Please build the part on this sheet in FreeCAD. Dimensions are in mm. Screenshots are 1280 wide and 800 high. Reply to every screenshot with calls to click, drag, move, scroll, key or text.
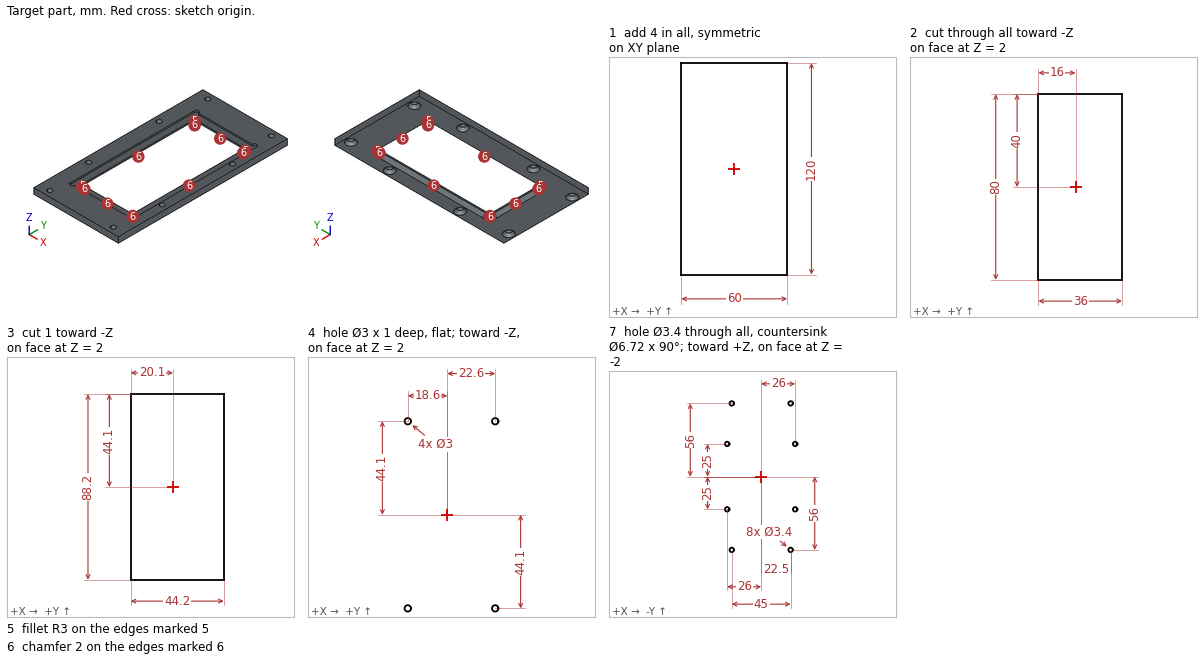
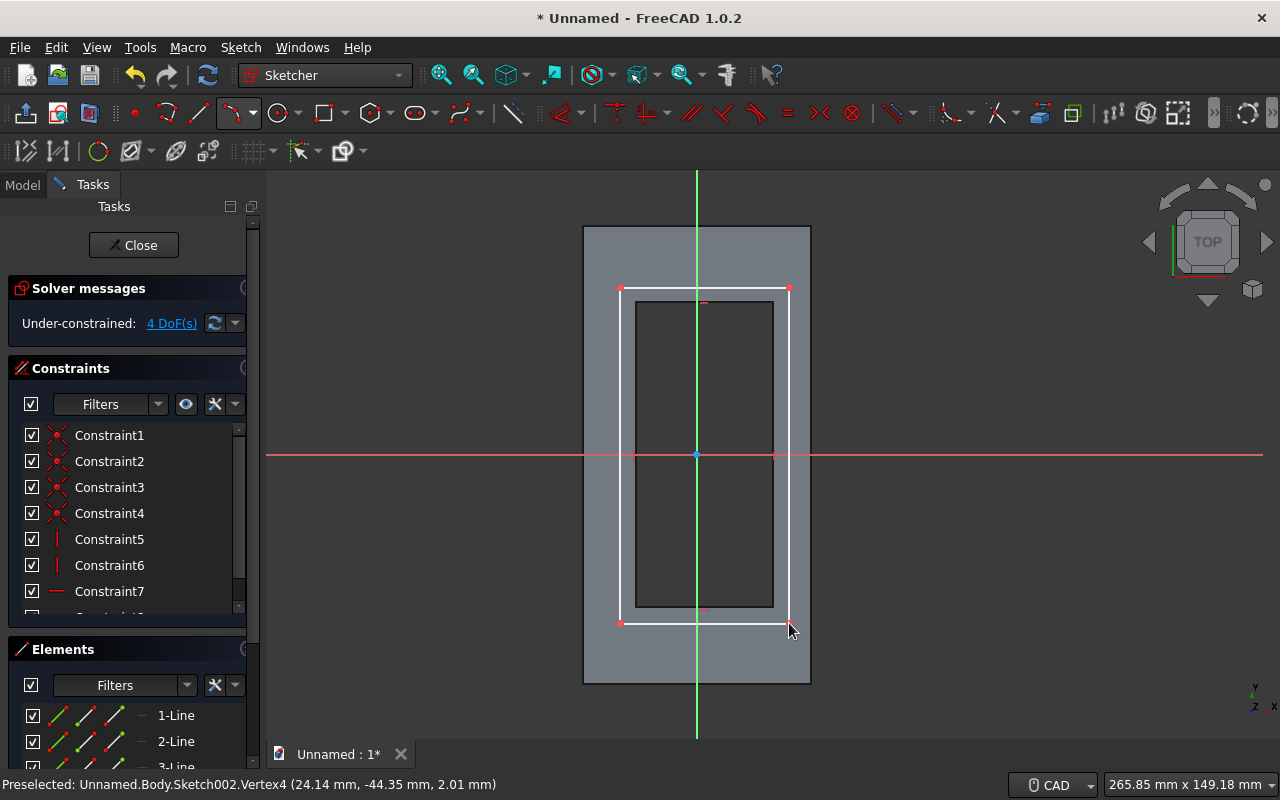
click(560, 114)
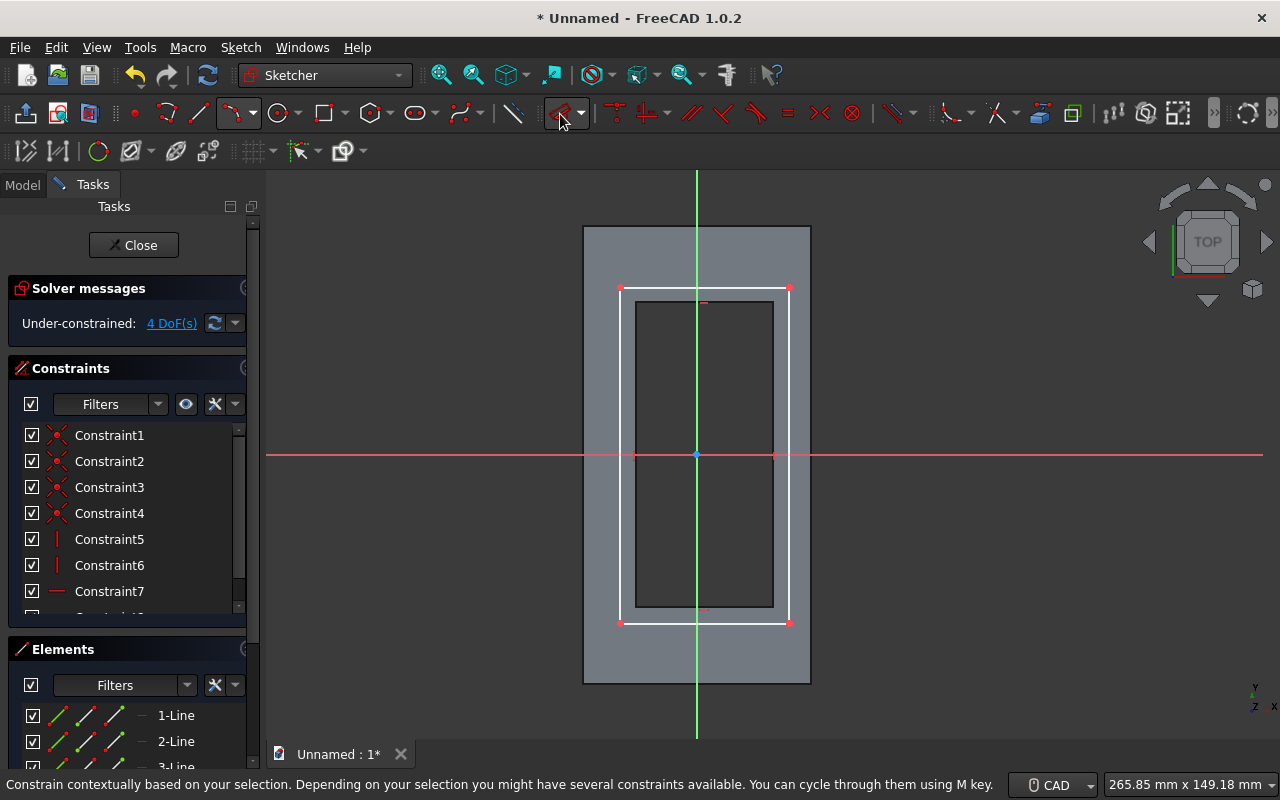
click(620, 389)
click(586, 379)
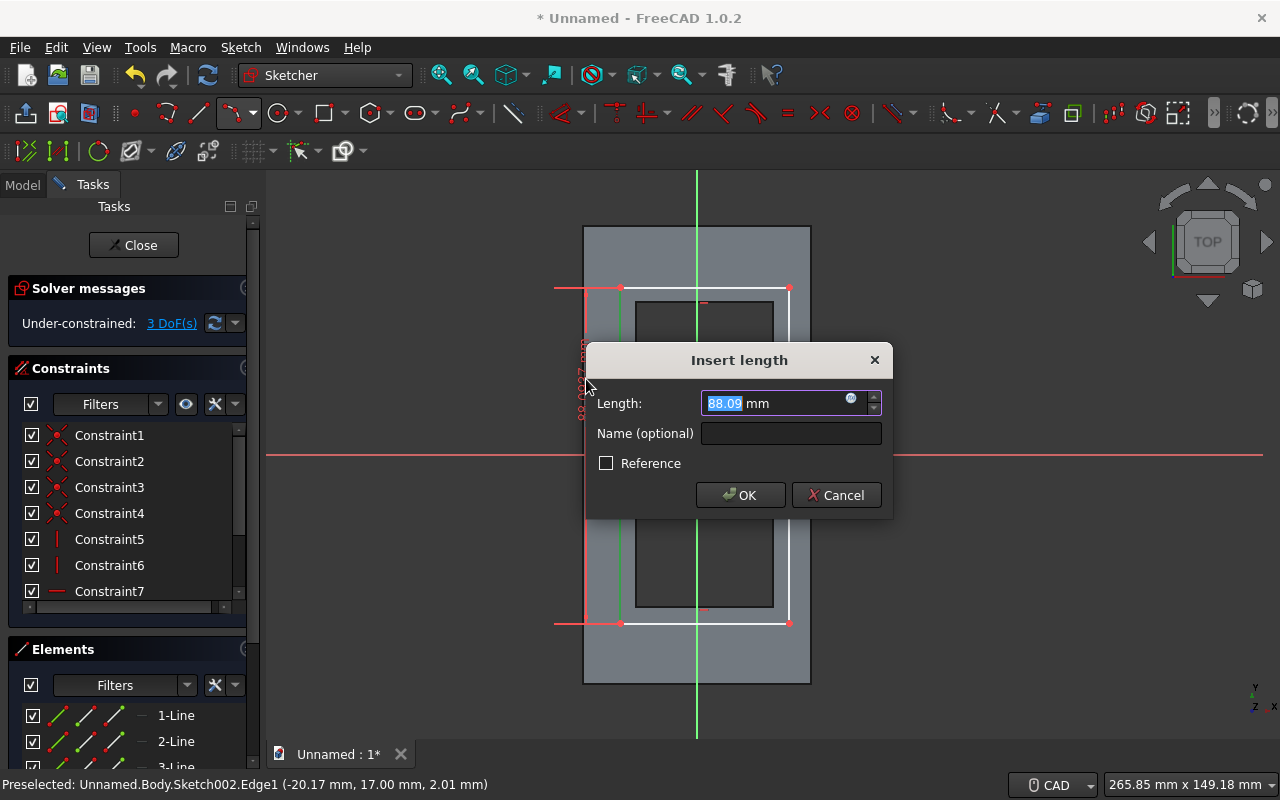
text(88.2)
key(Return)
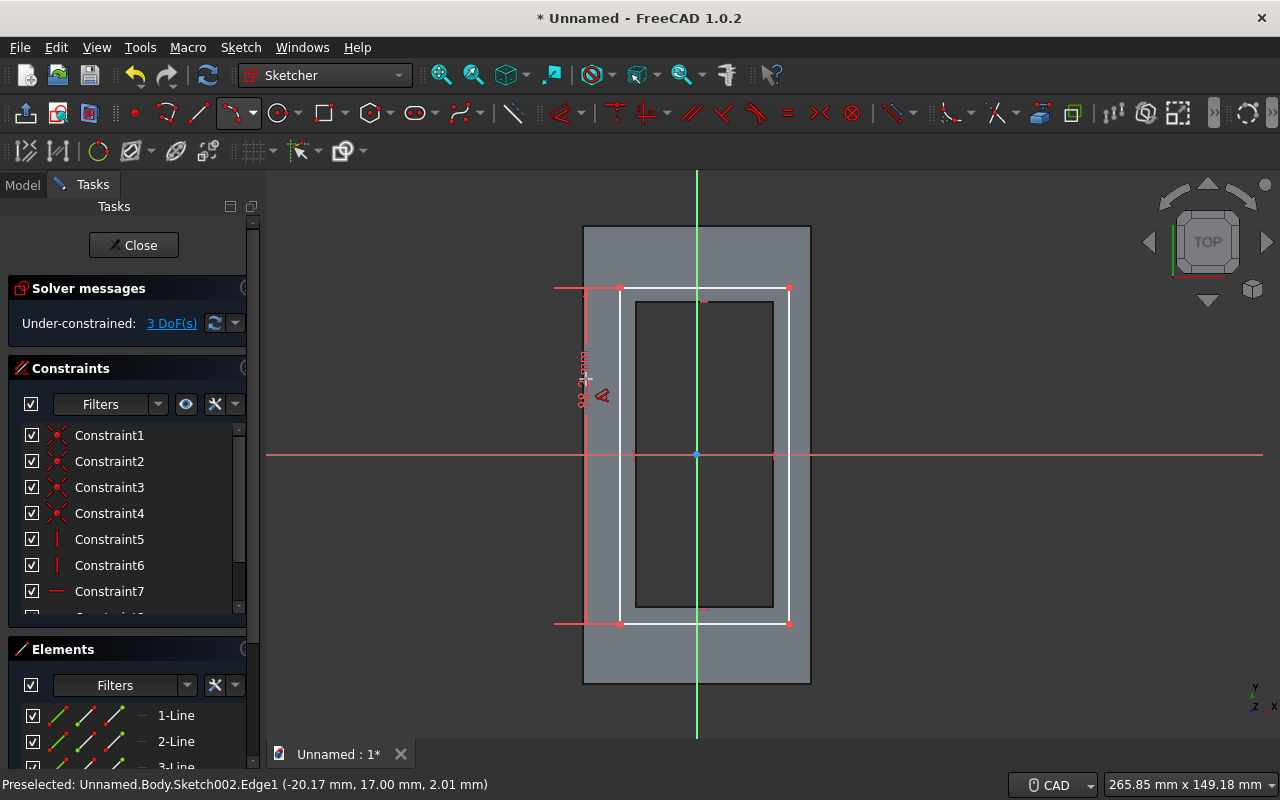
click(671, 624)
click(666, 658)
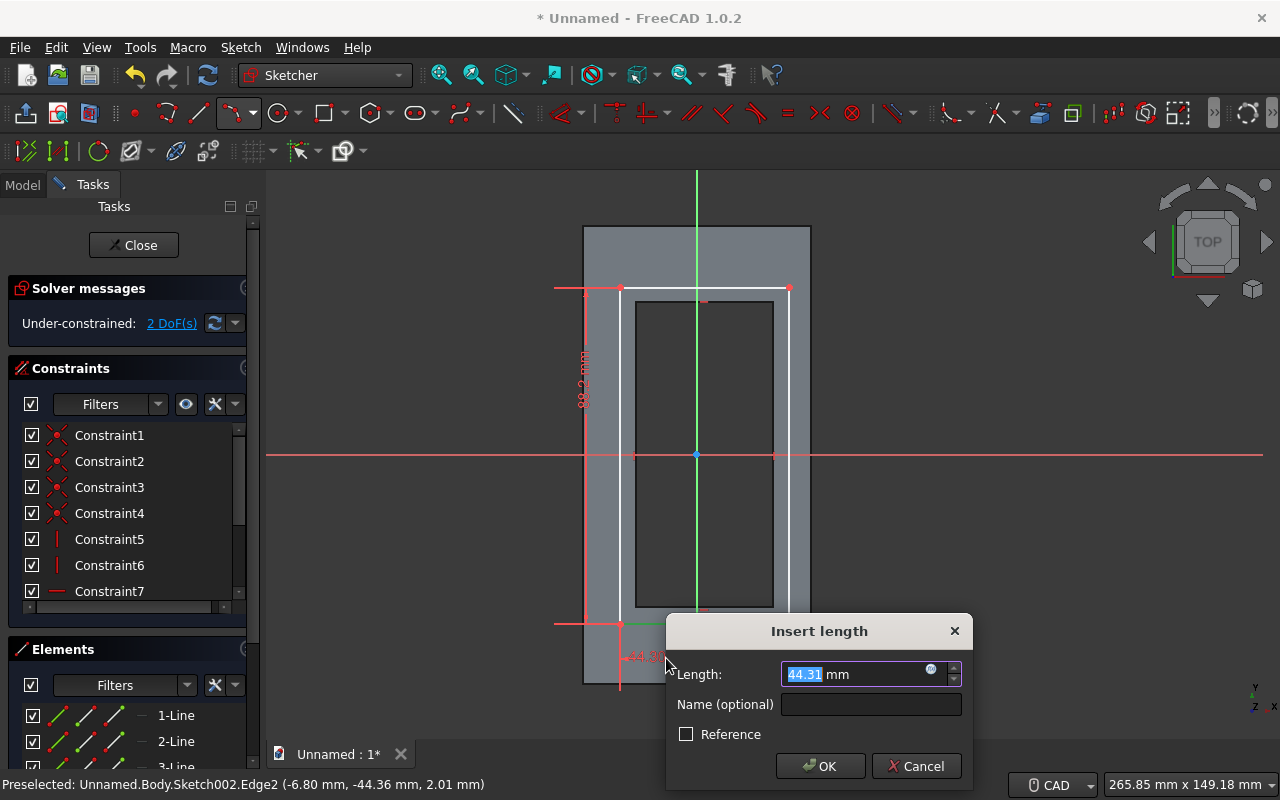
text(44.2)
key(Return)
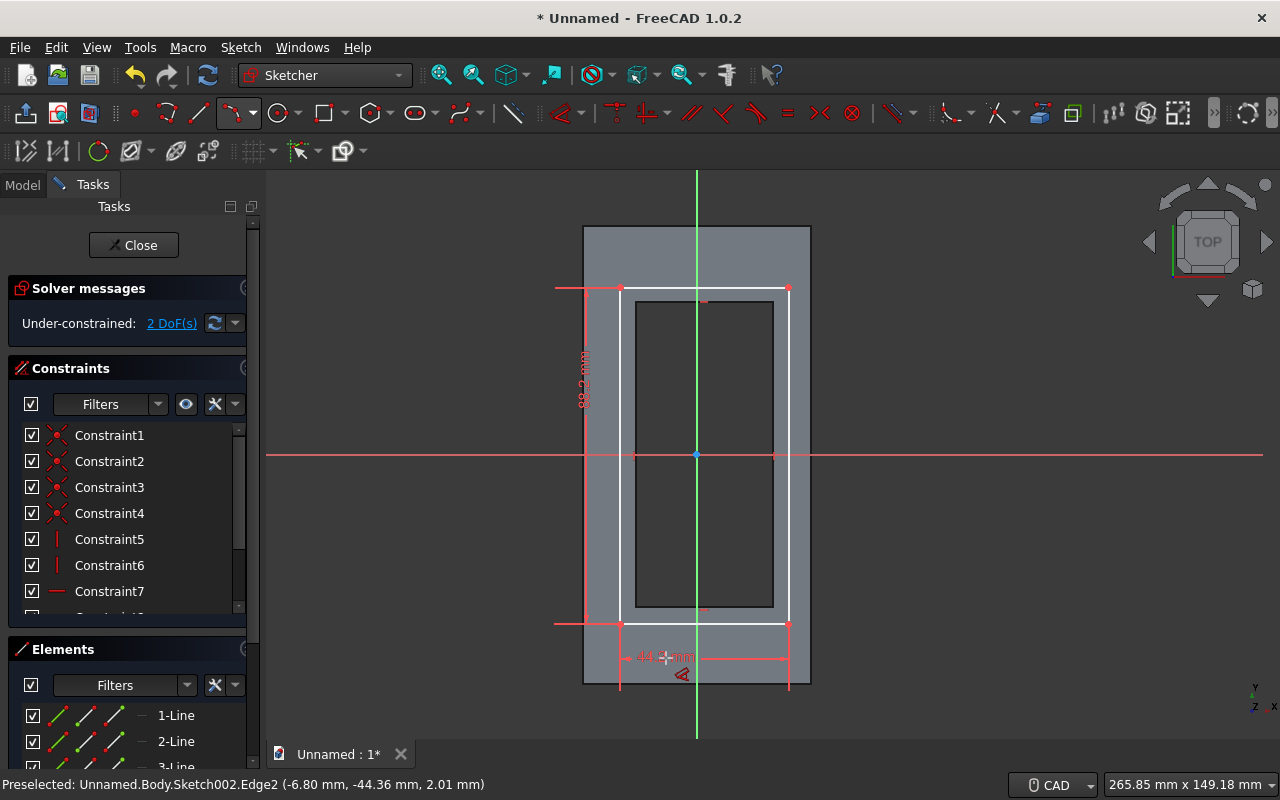
click(620, 288)
click(659, 254)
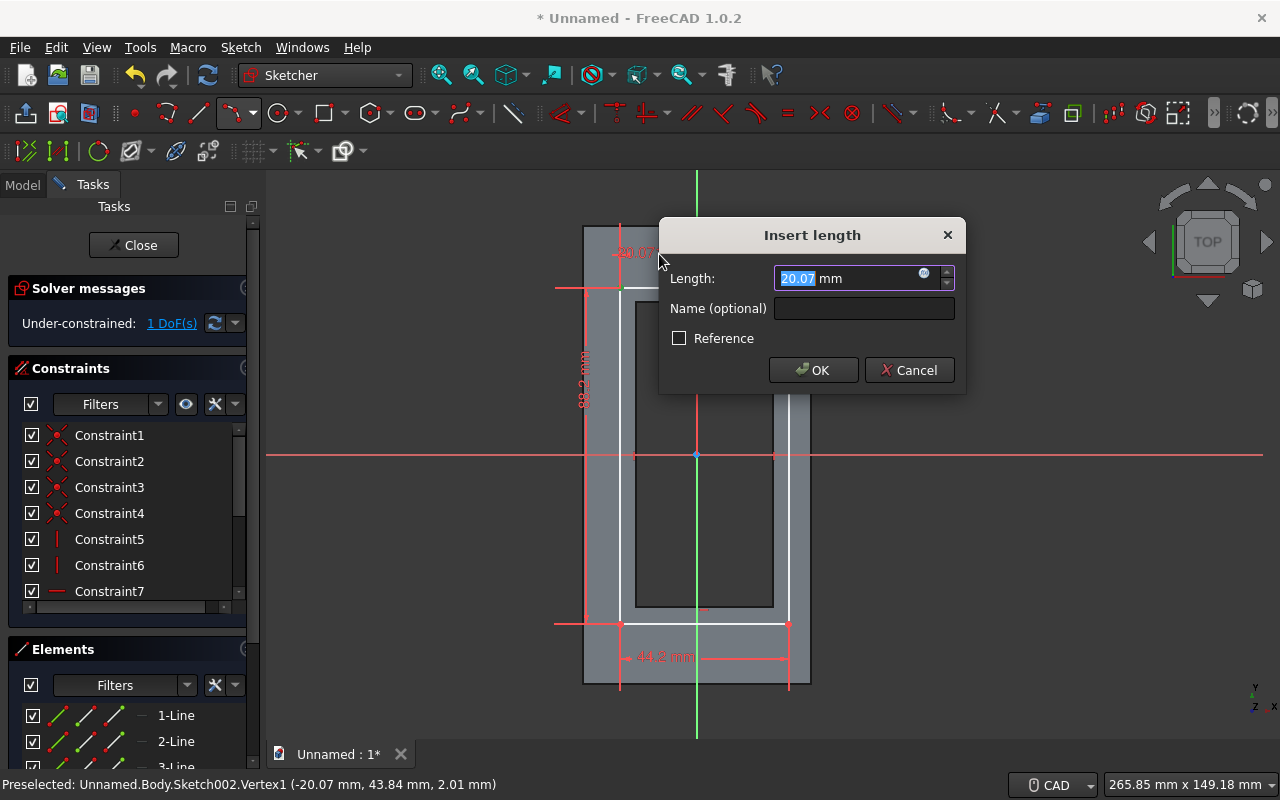
text(20.1)
key(Return)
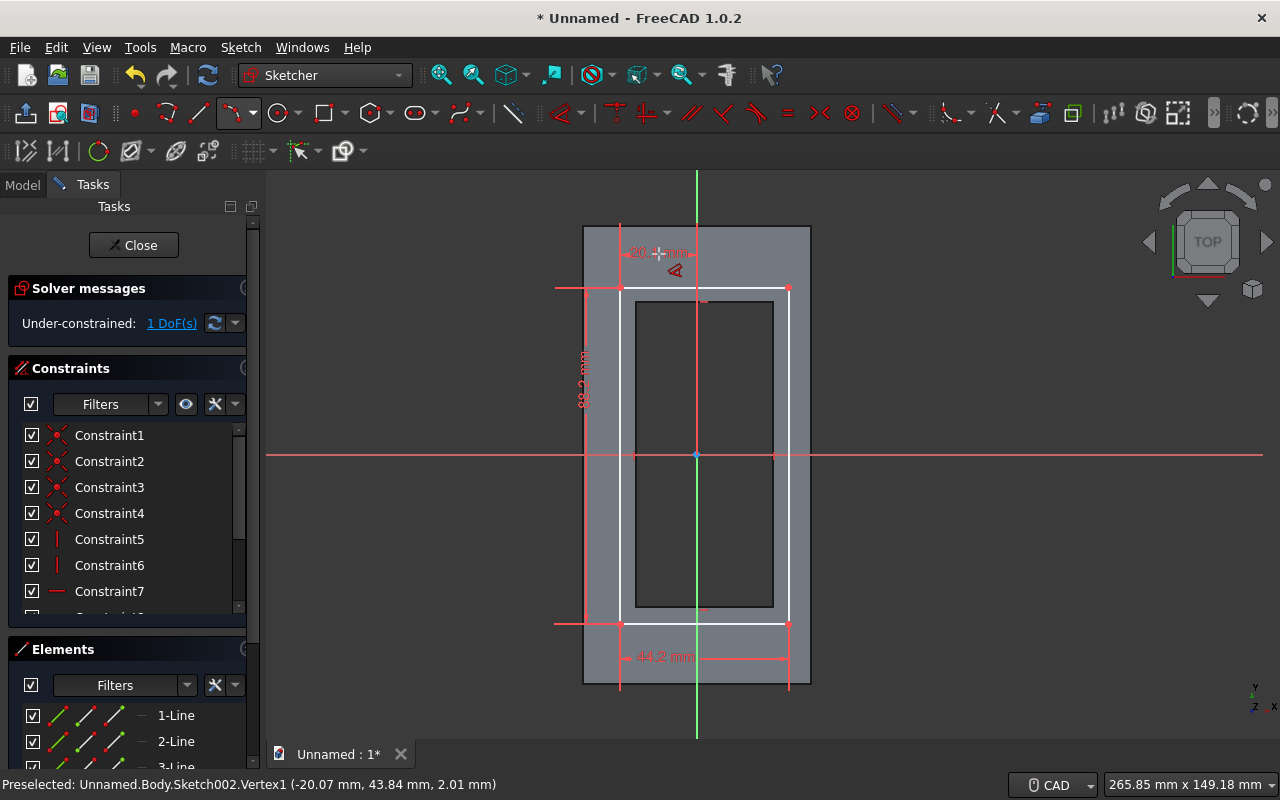
click(620, 288)
click(586, 333)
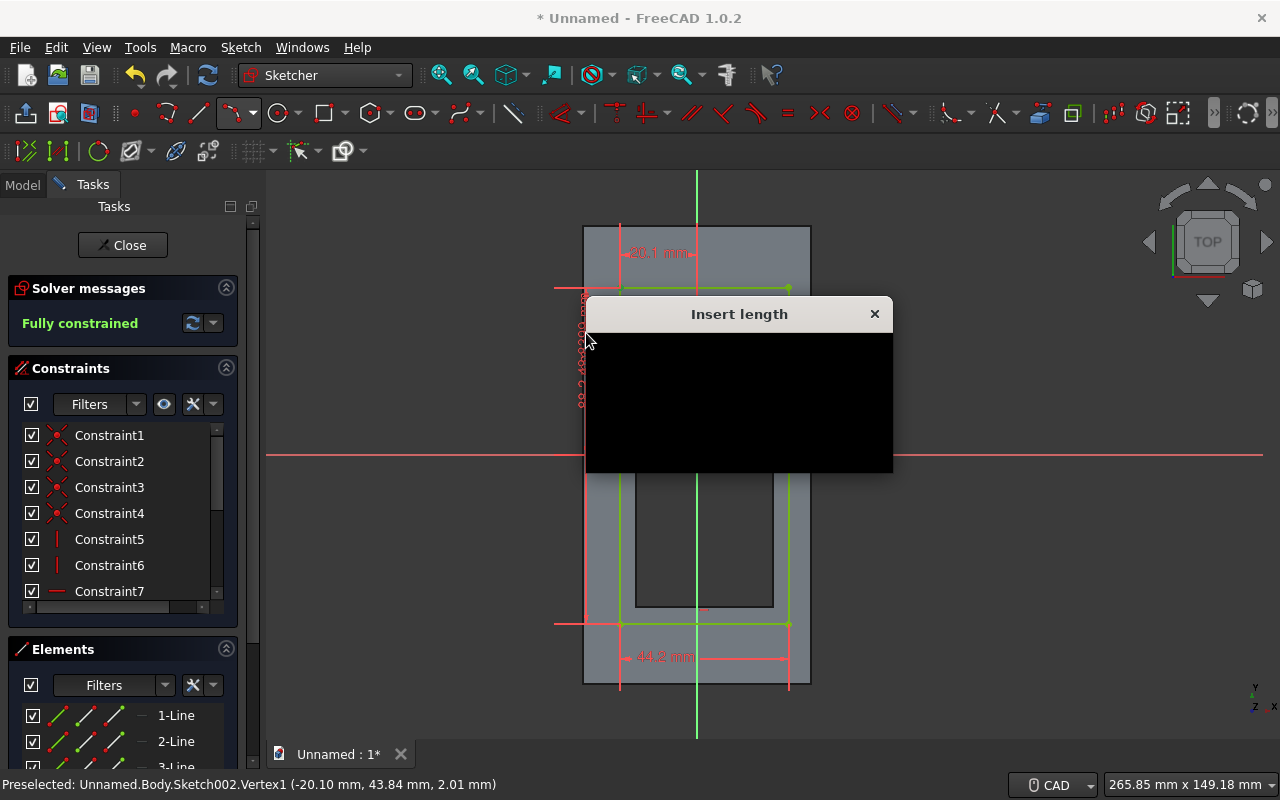
text(44.1)
key(Return)
key(Escape)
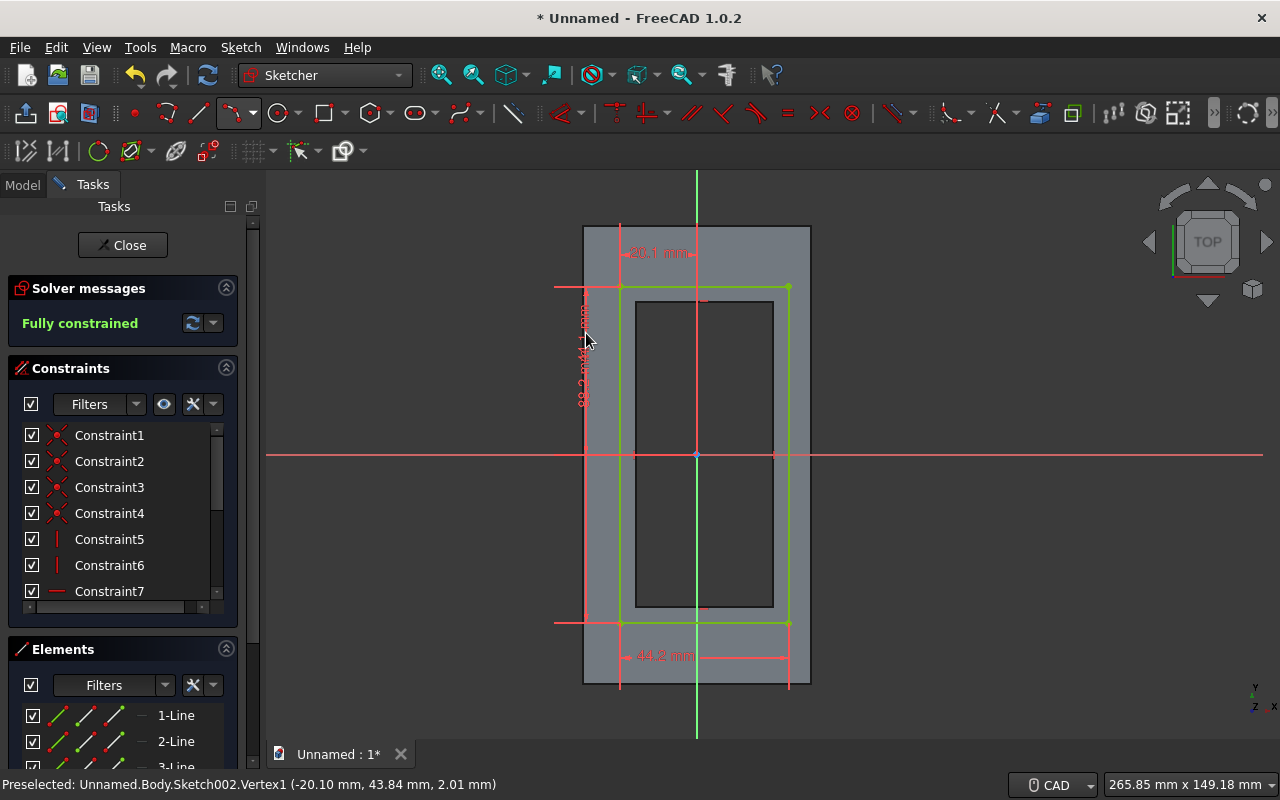
click(123, 245)